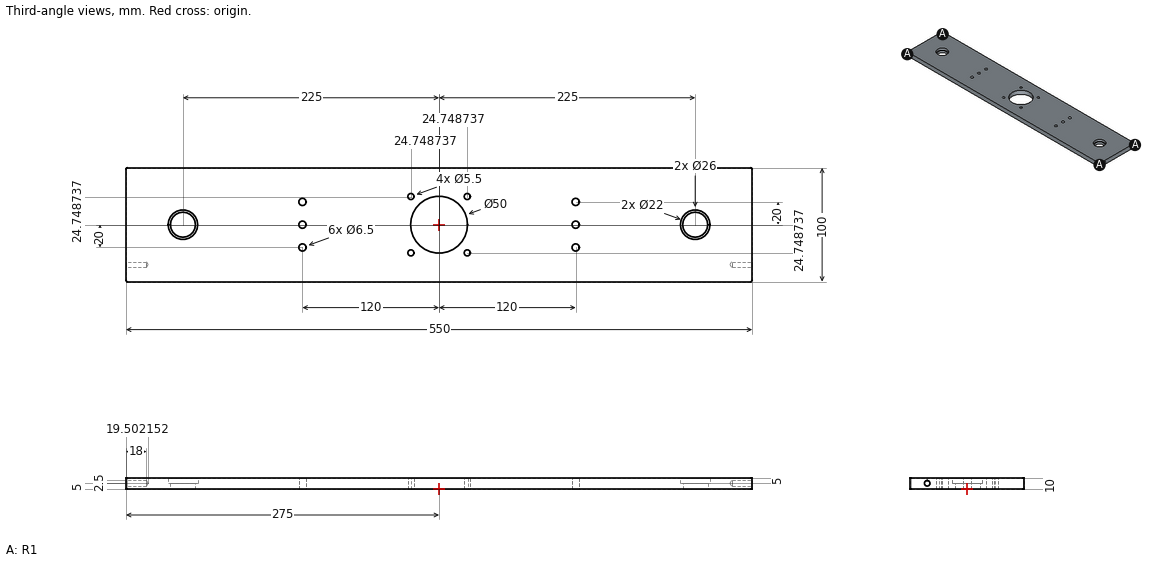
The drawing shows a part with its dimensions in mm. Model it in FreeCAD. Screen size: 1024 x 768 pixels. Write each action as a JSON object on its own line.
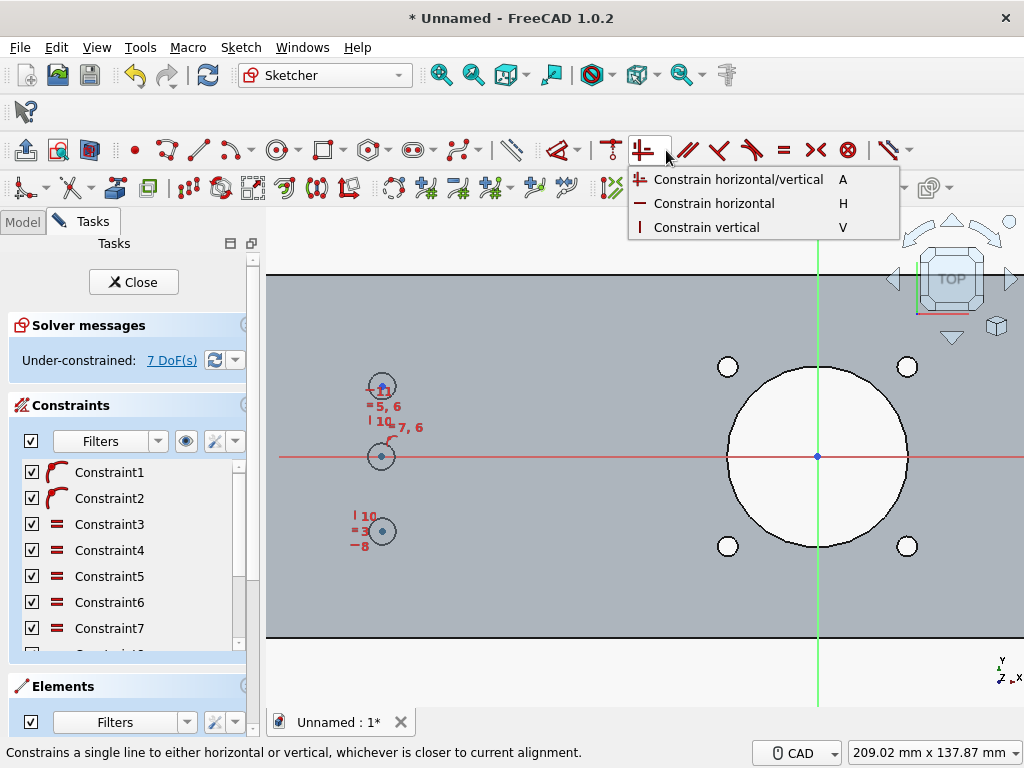
{"action": "left_click", "coordinate": [764, 227]}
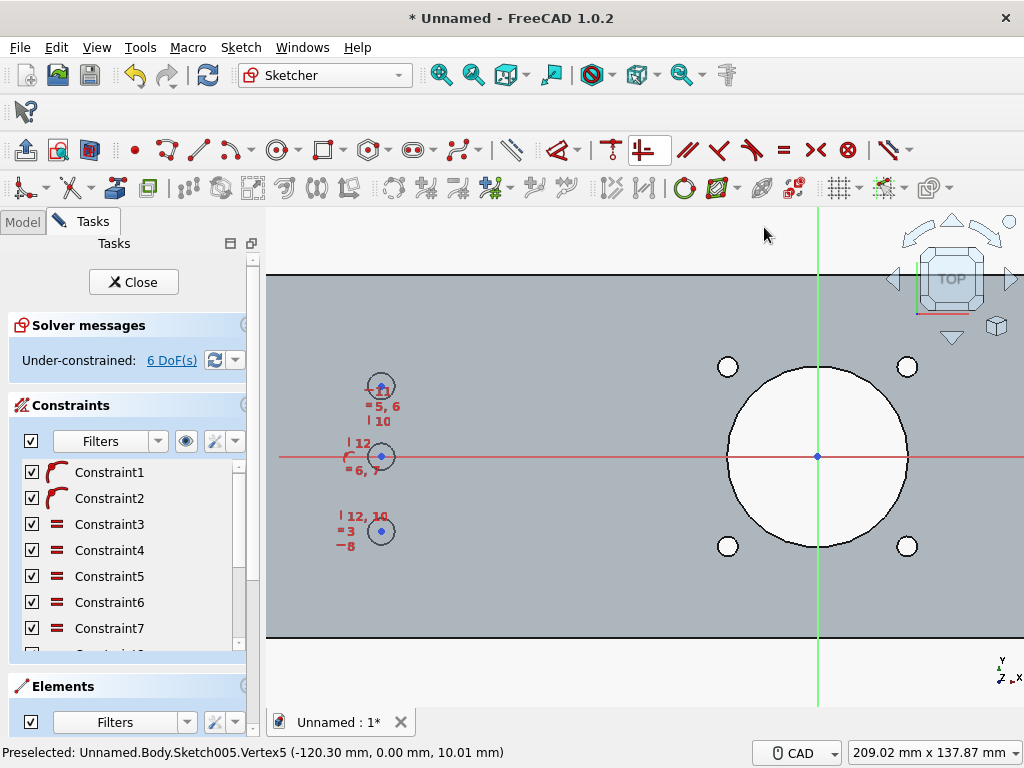
{"action": "scroll", "coordinate": [380, 457], "scroll_direction": "down", "scroll_amount": 4}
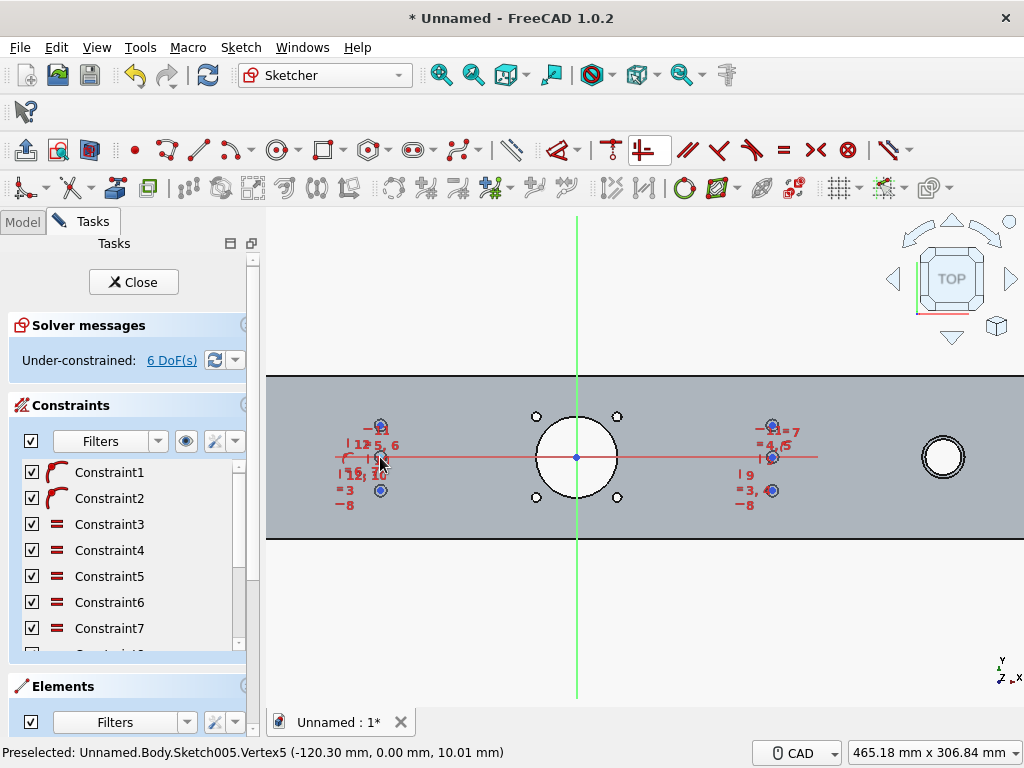
{"action": "left_click", "coordinate": [772, 491]}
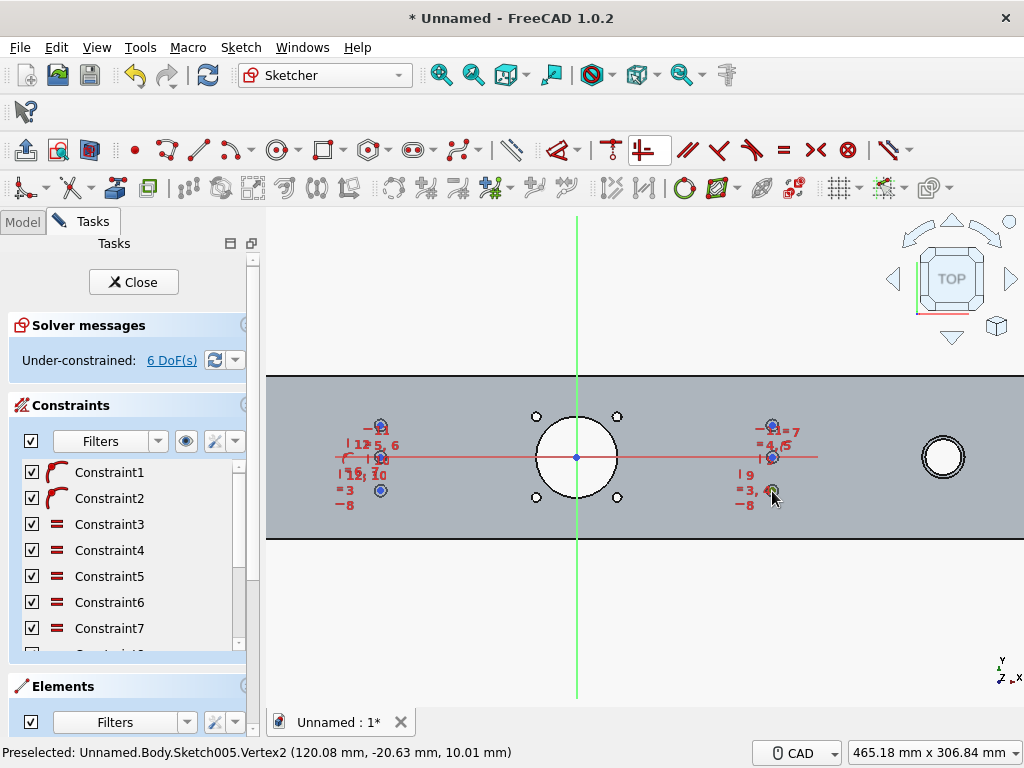
{"action": "left_click", "coordinate": [773, 457]}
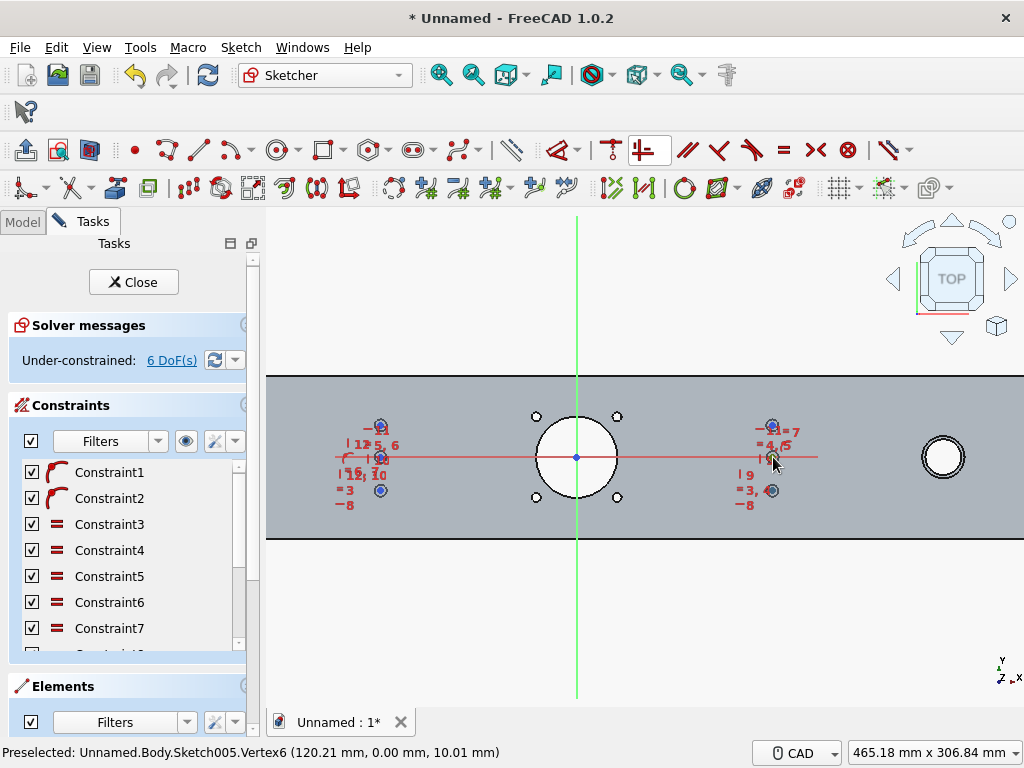
{"action": "key", "text": "v"}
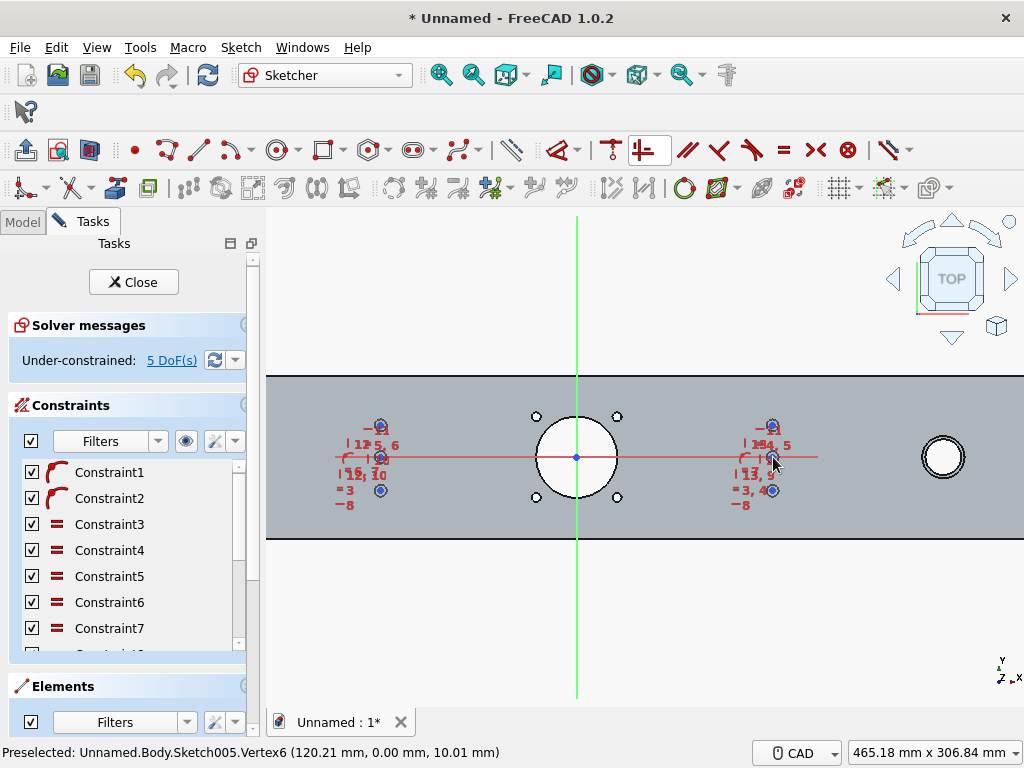
{"action": "key", "text": "d"}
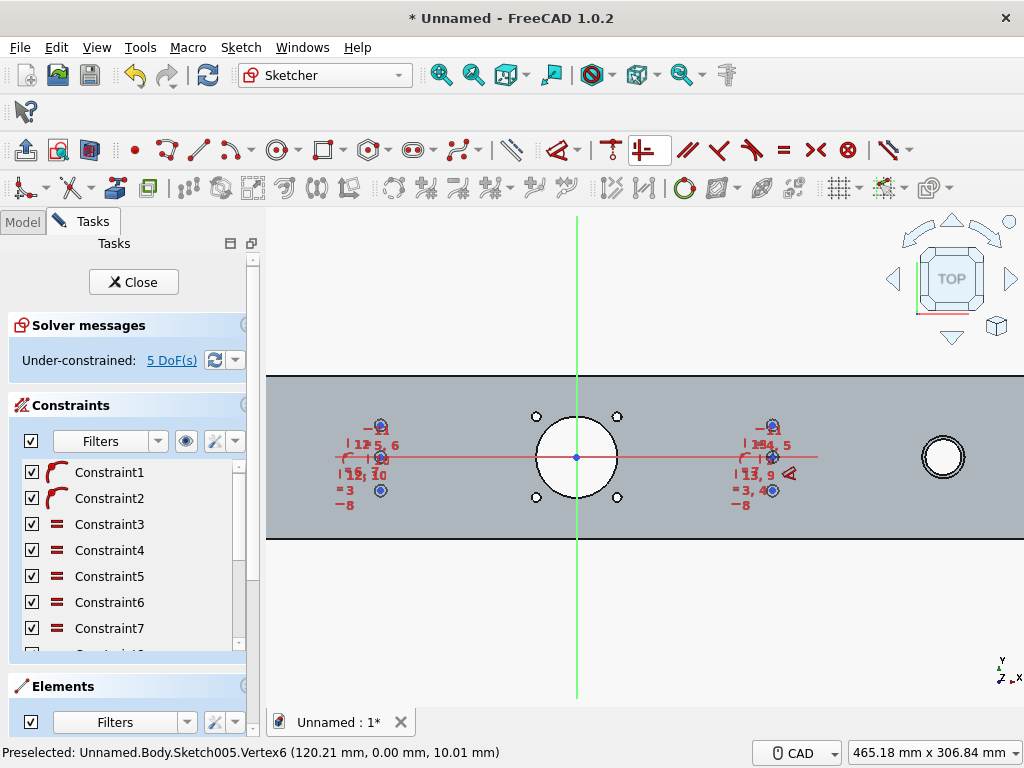
{"action": "scroll", "coordinate": [385, 487], "scroll_direction": "up", "scroll_amount": 7}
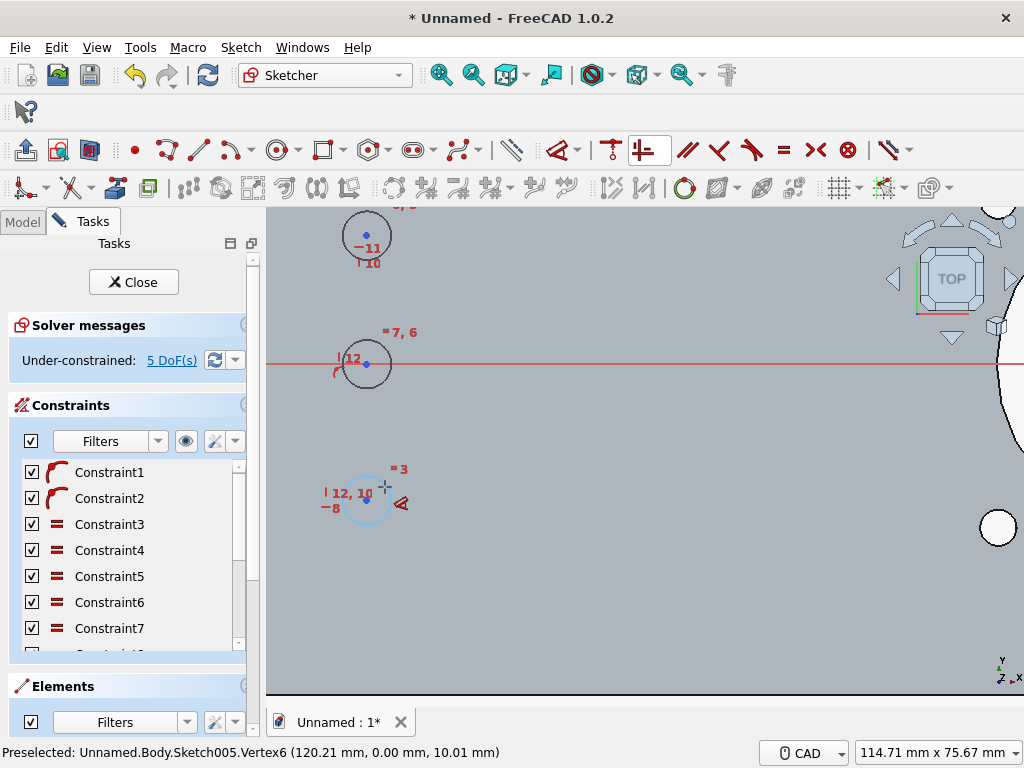
{"action": "left_click", "coordinate": [384, 483]}
{"action": "left_click", "coordinate": [406, 460]}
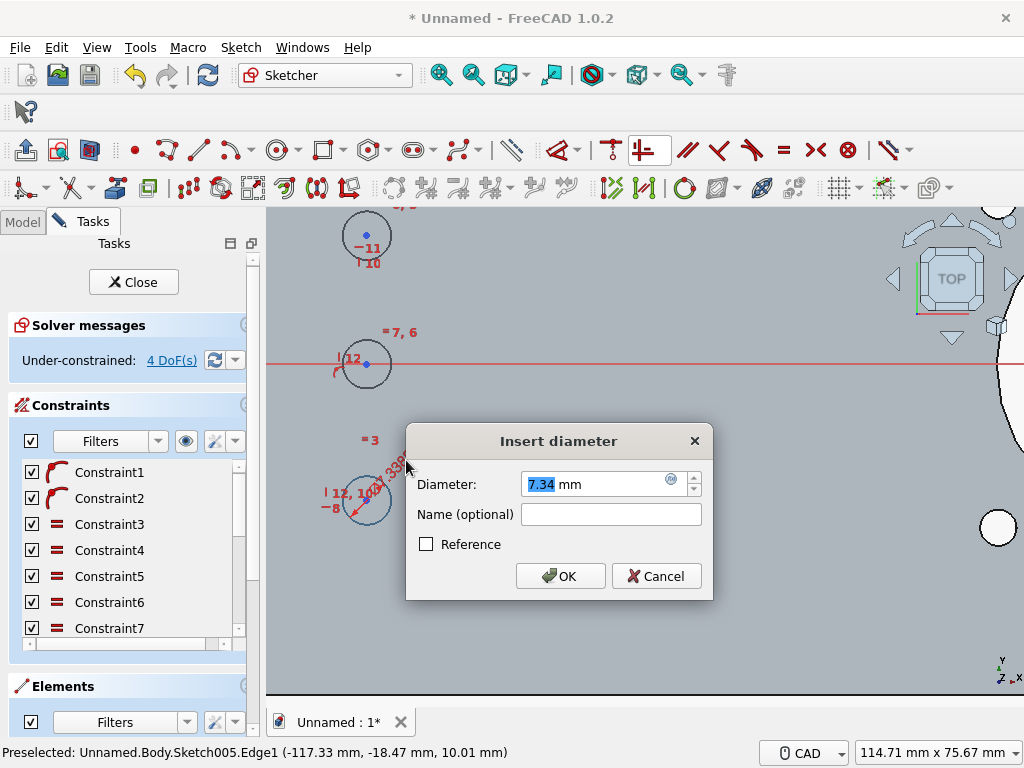
{"action": "type", "text": "6.5"}
{"action": "key", "text": "Return"}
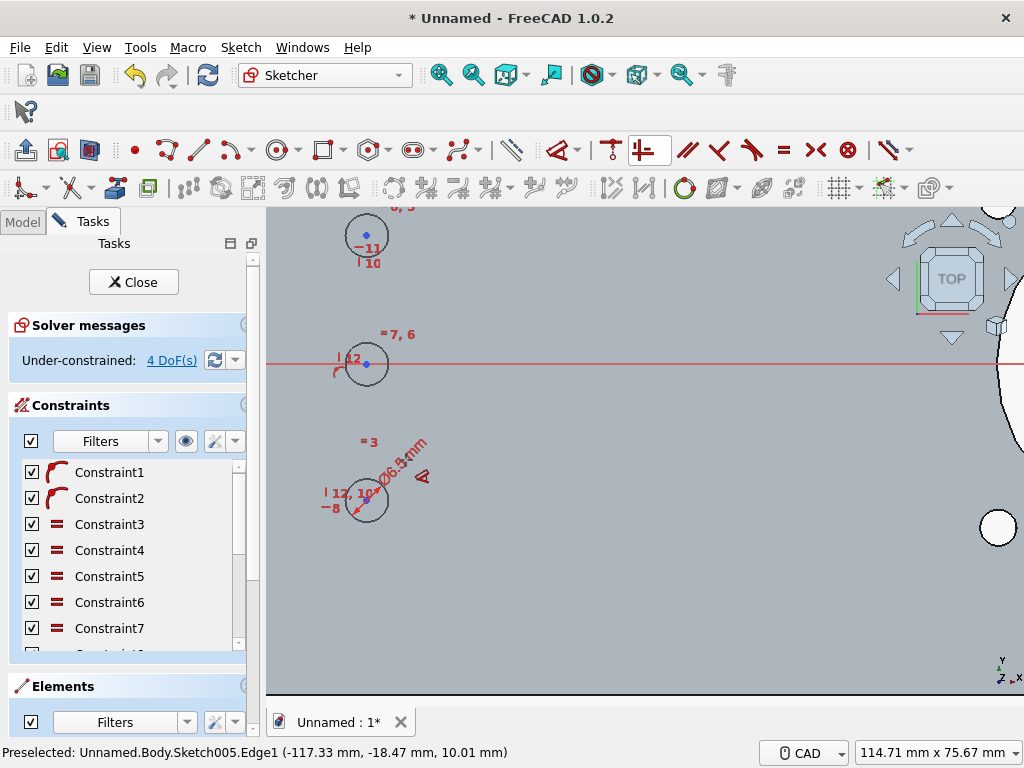
{"action": "scroll", "coordinate": [385, 487], "scroll_direction": "down", "scroll_amount": 7}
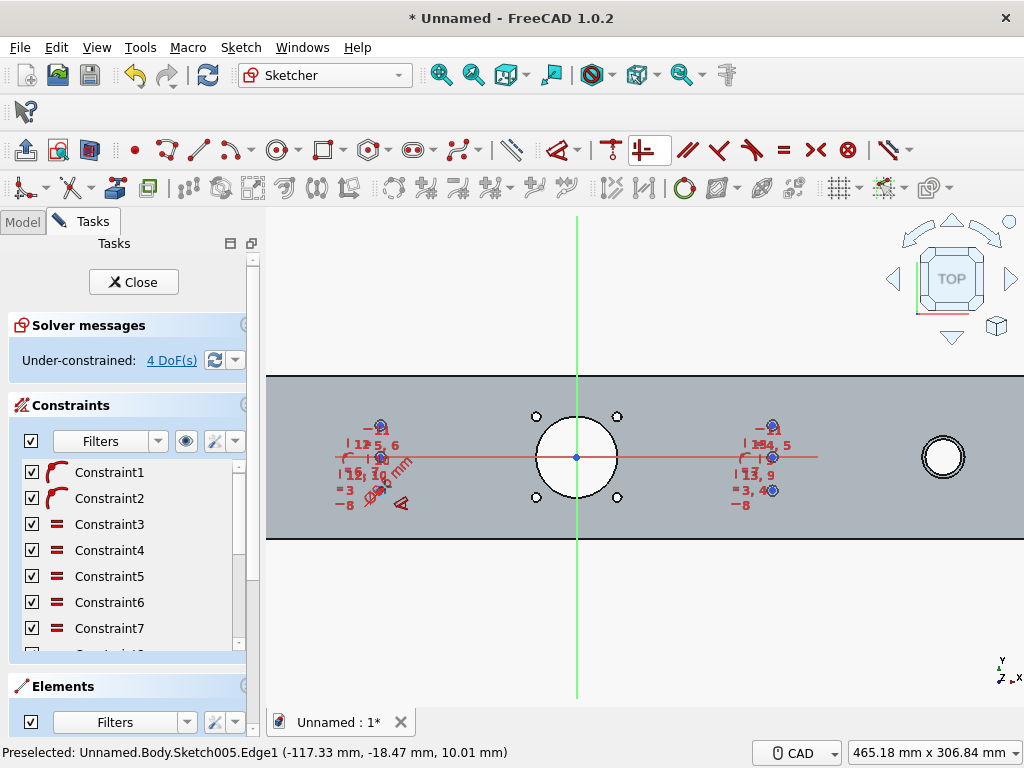
{"action": "left_click", "coordinate": [381, 491]}
{"action": "left_click", "coordinate": [611, 474]}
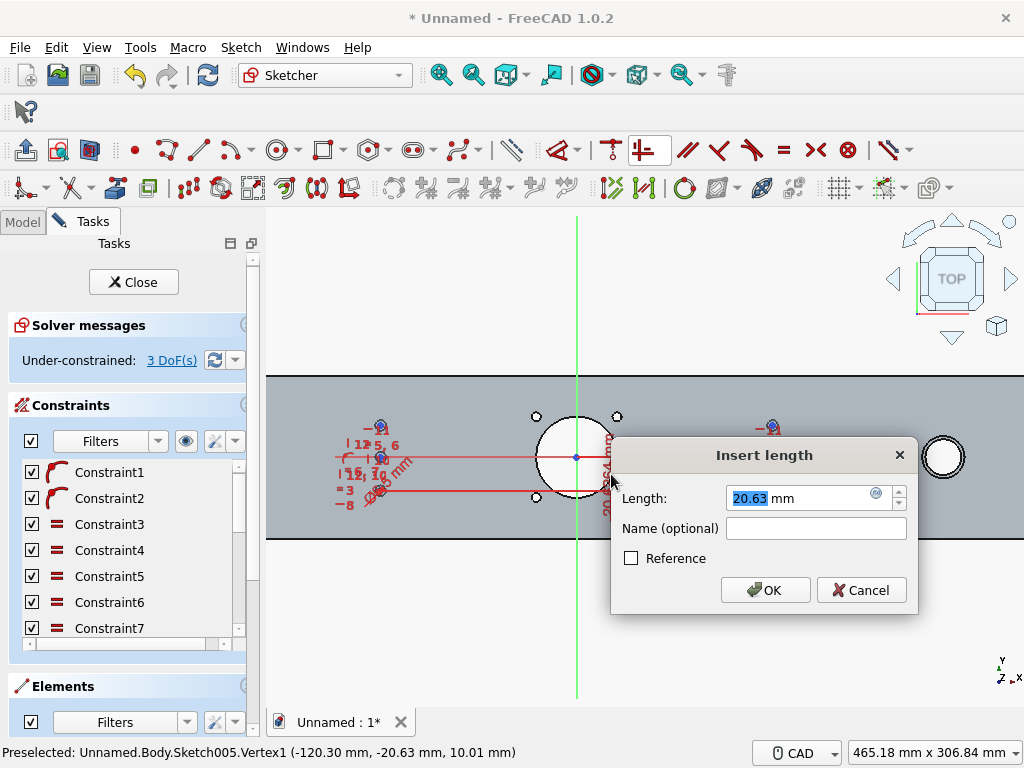
{"action": "type", "text": "20"}
{"action": "key", "text": "Return"}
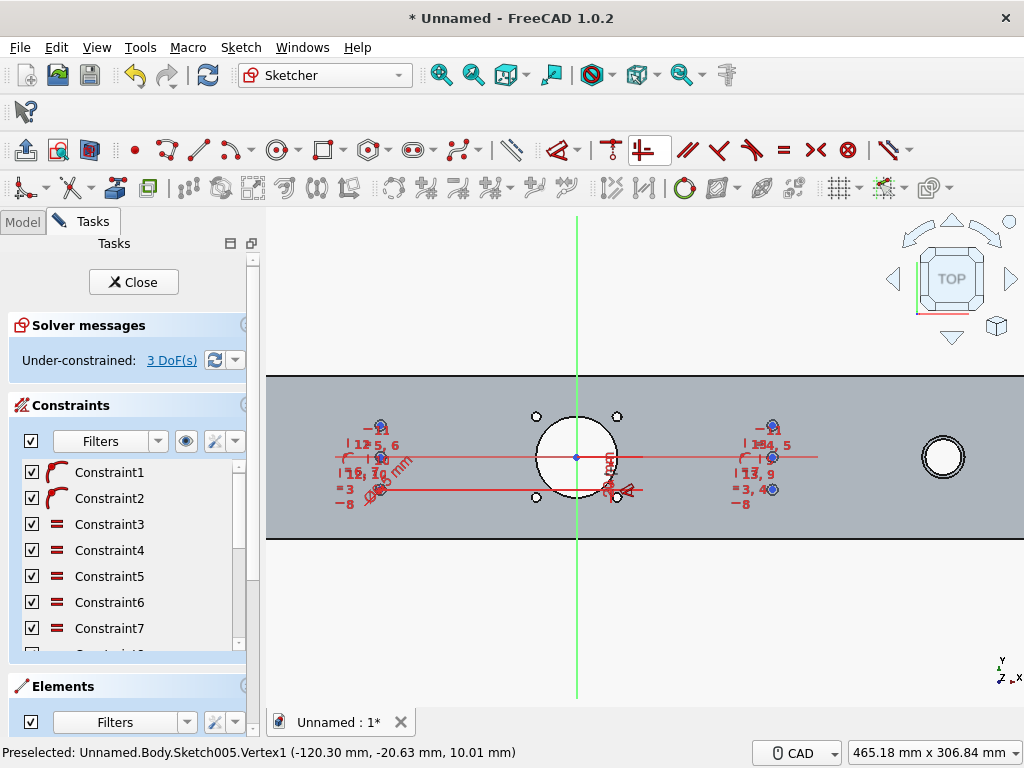
{"action": "left_click", "coordinate": [773, 425]}
{"action": "left_click", "coordinate": [807, 441]}